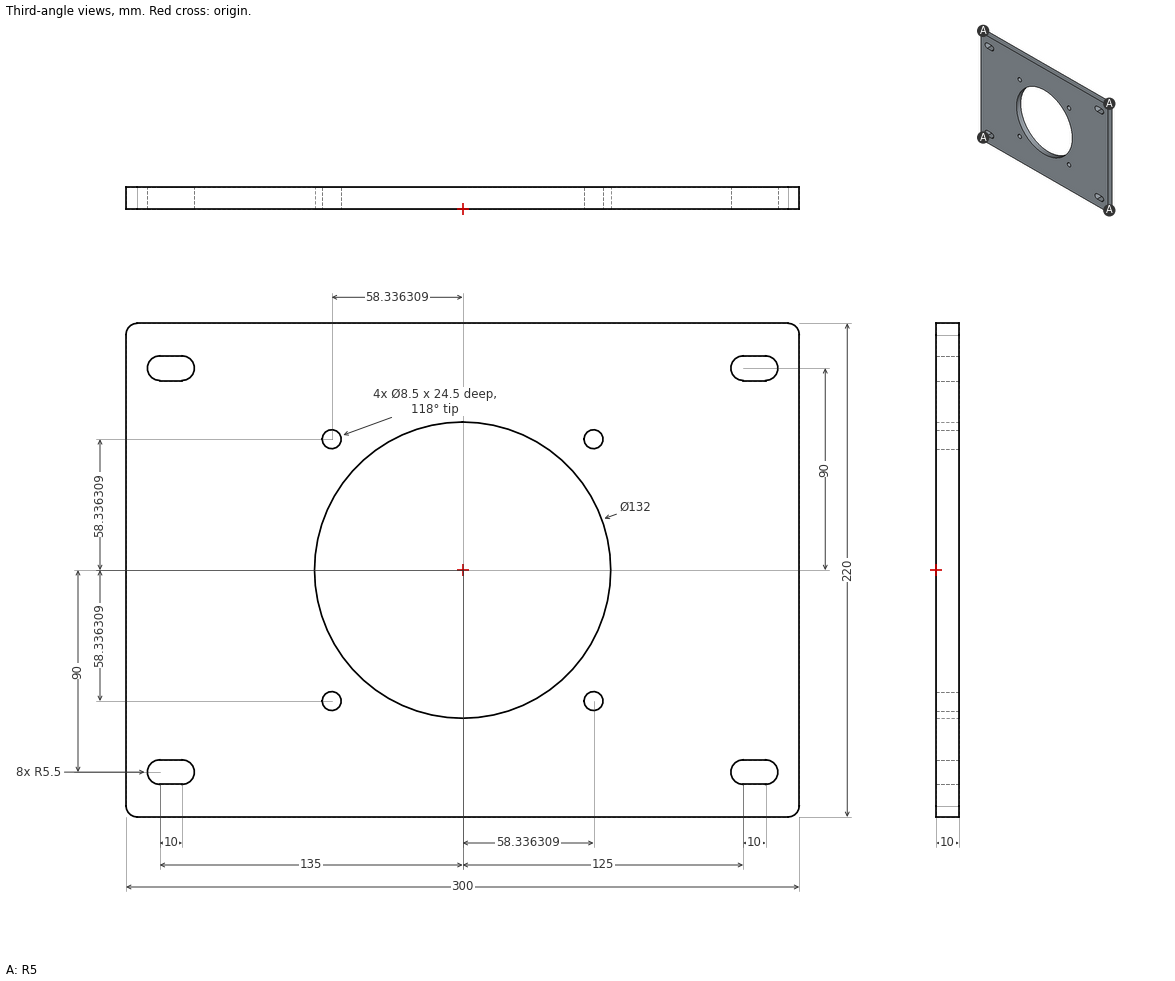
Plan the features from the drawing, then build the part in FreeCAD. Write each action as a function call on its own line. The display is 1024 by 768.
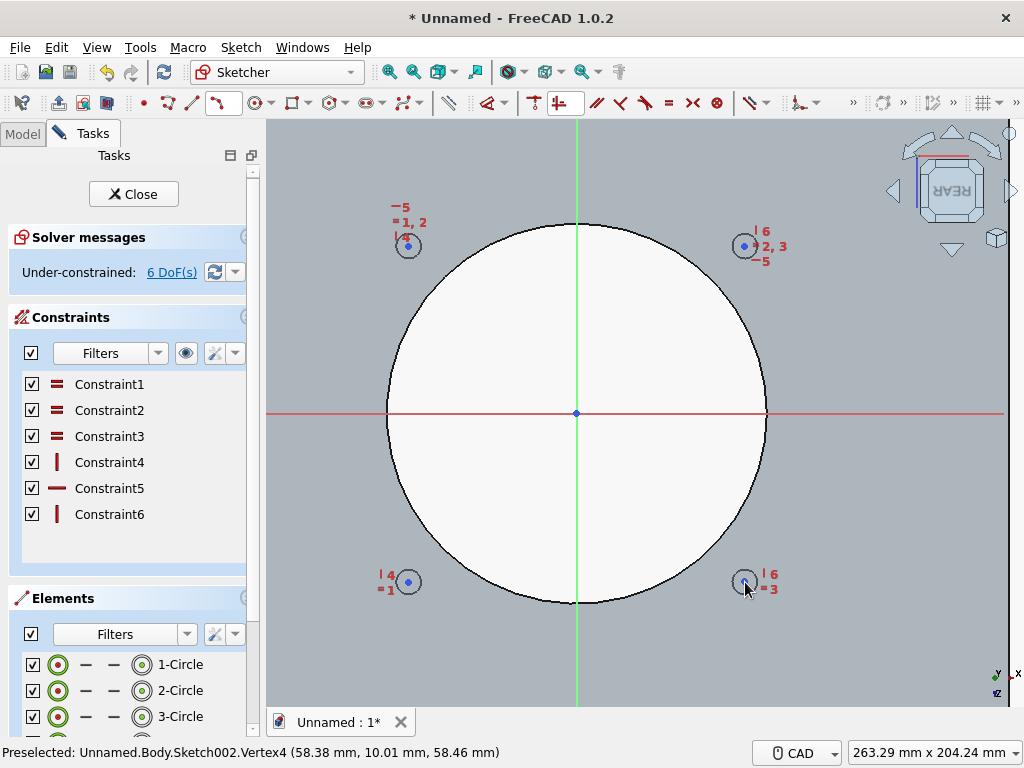
click(409, 582)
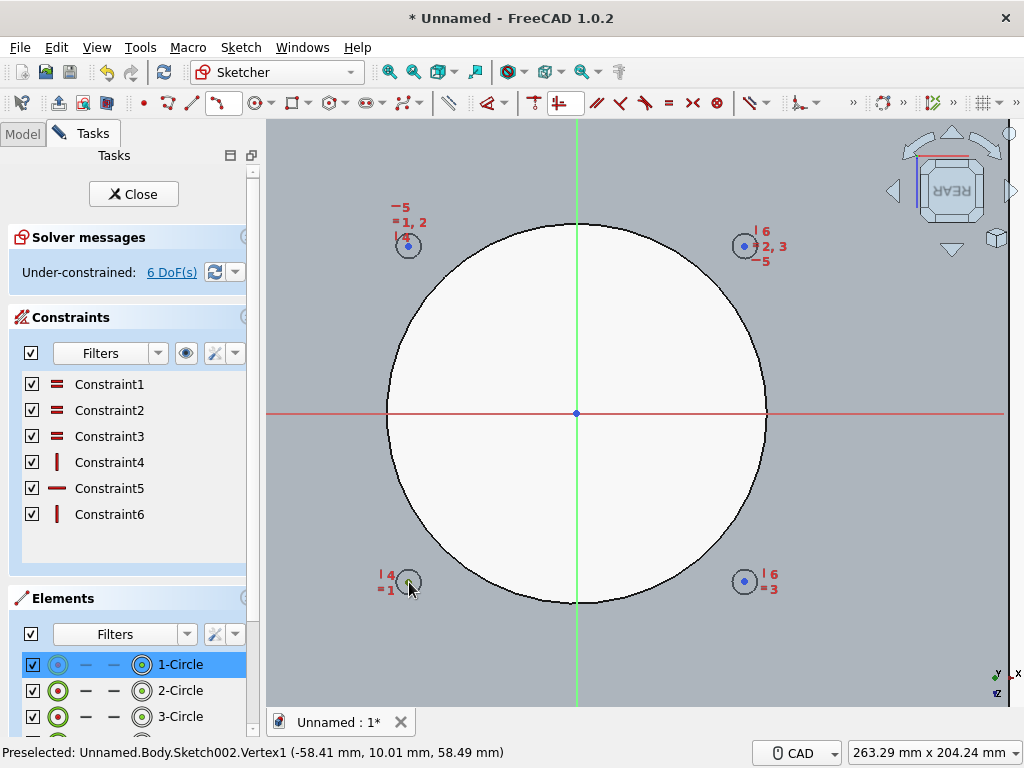
click(745, 582)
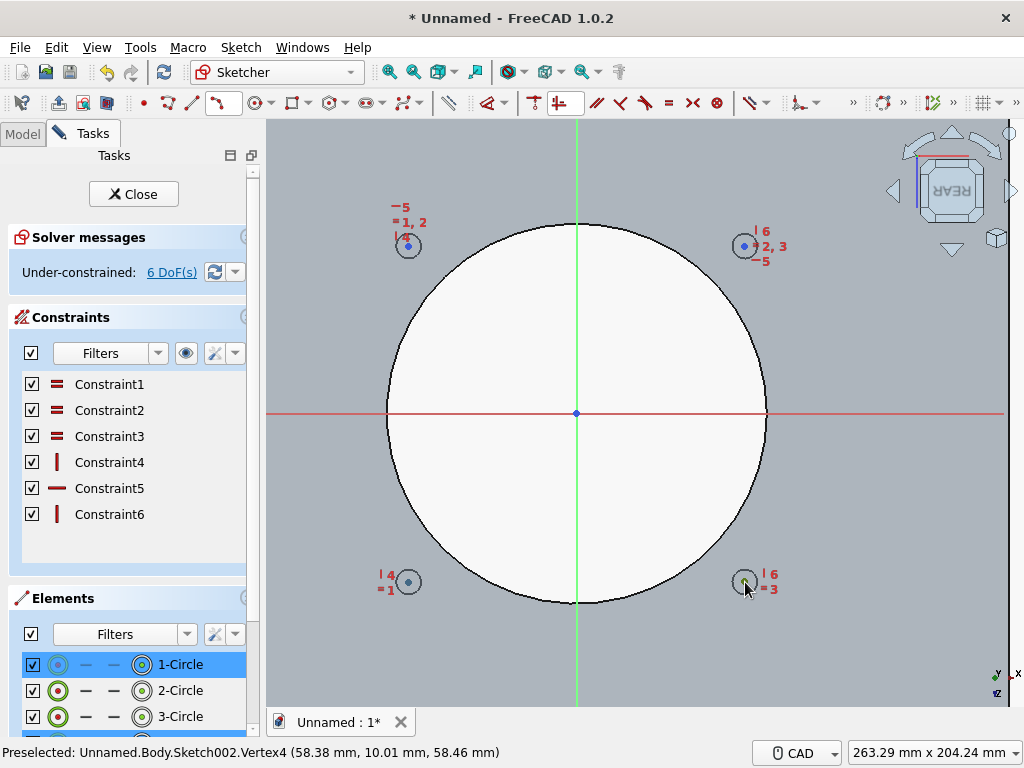
key(h)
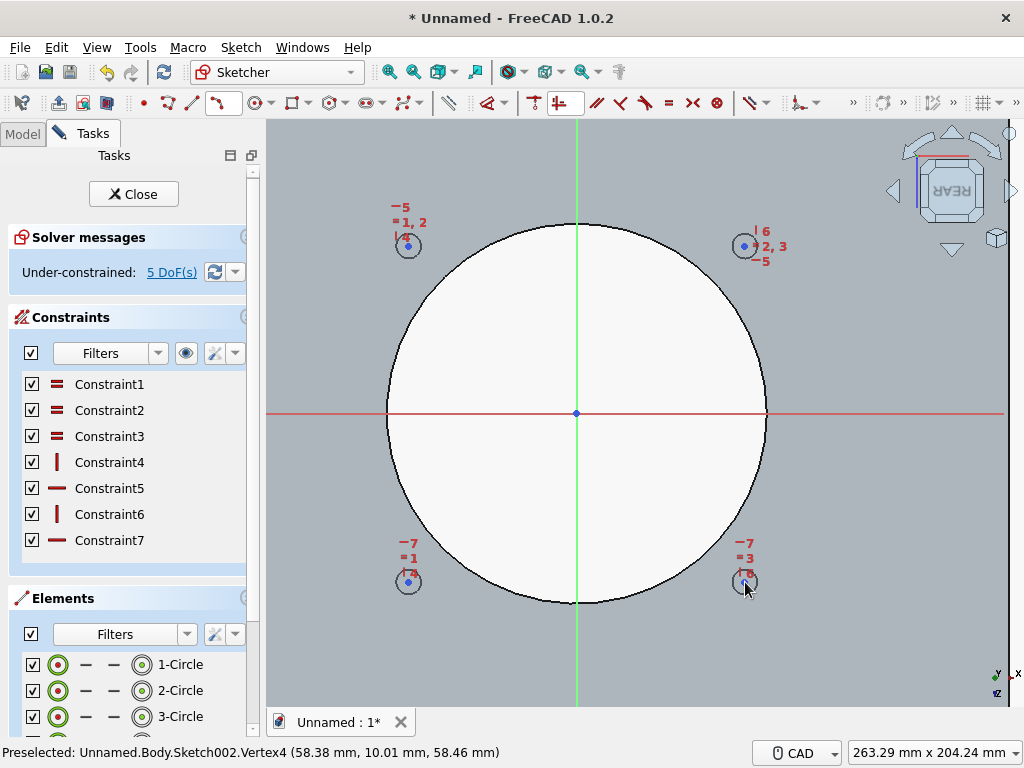
key(d)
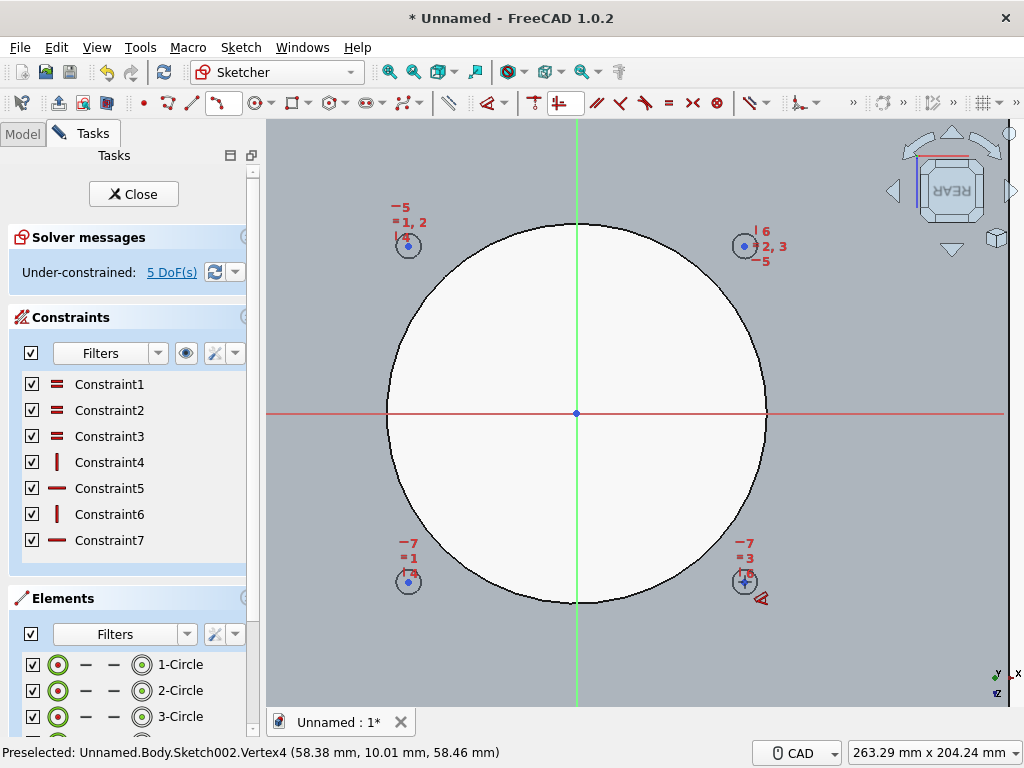
scroll(417, 573, up, 3)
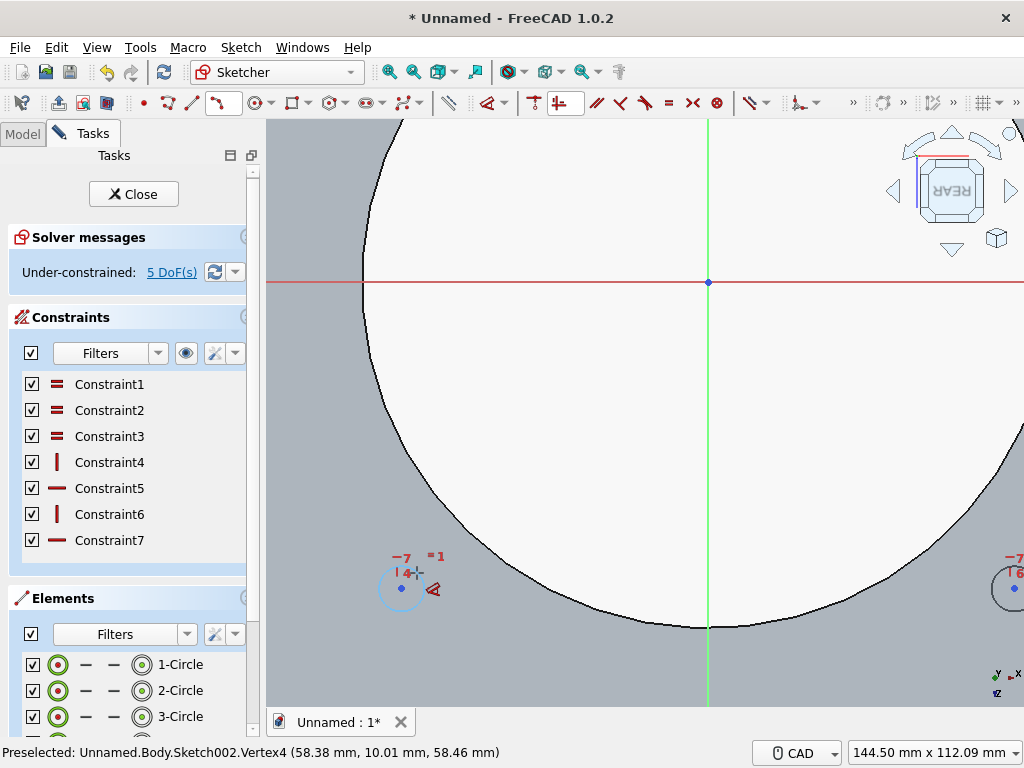
click(418, 573)
click(441, 551)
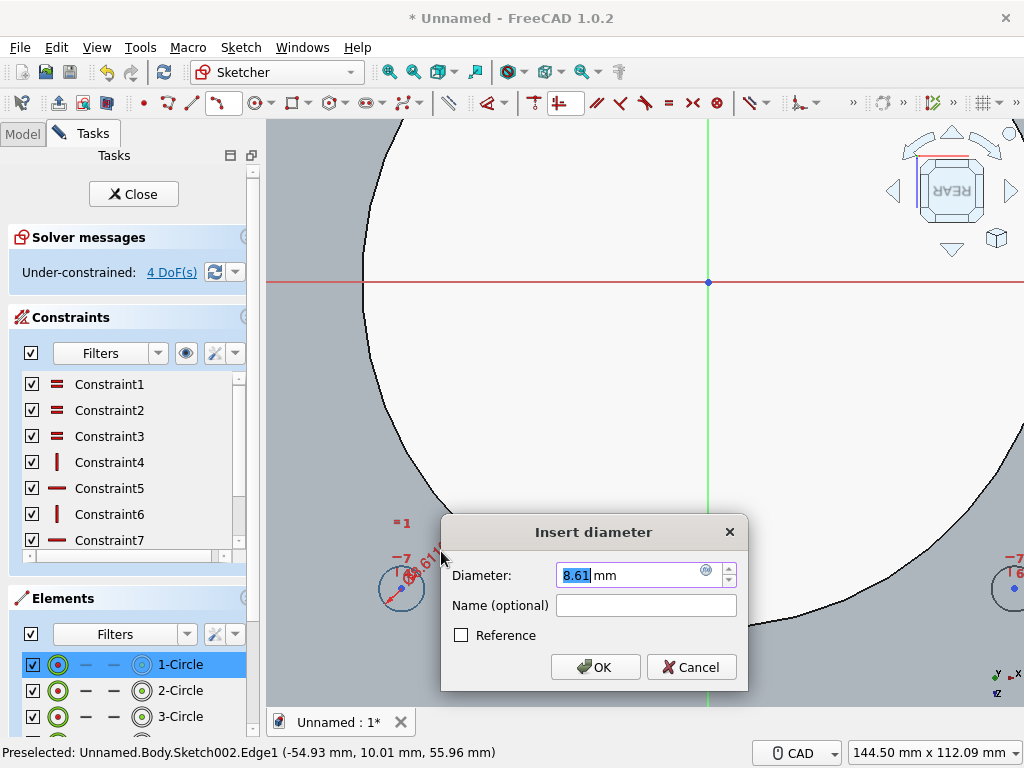
text(8.5)
key(Return)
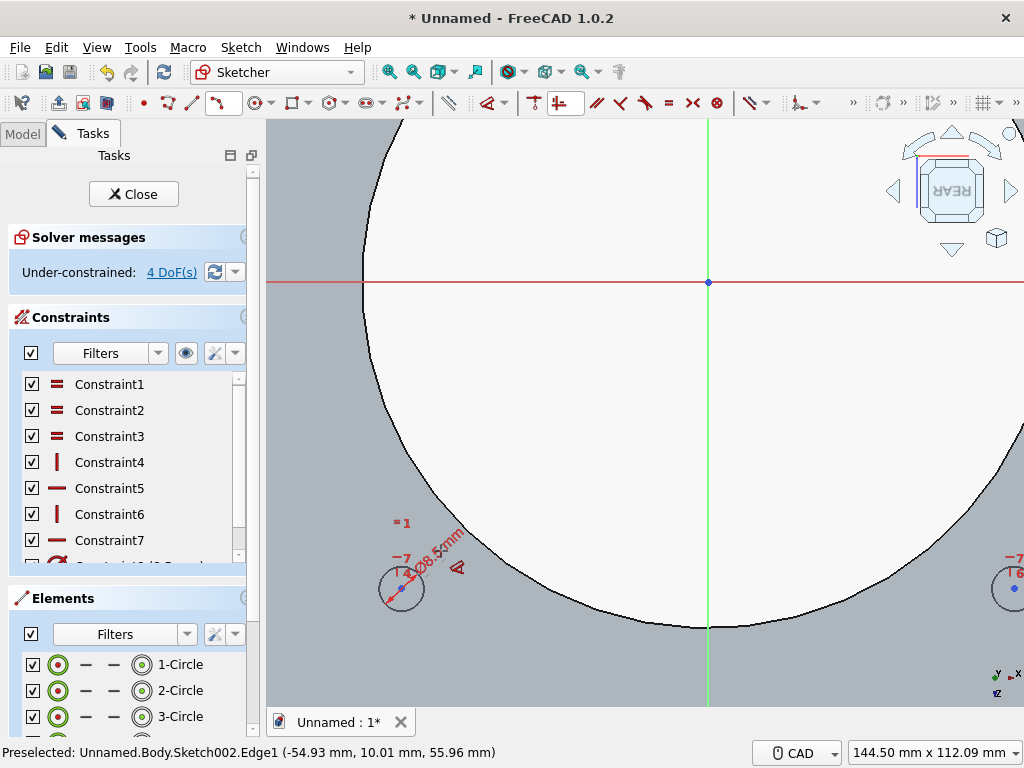
click(402, 589)
click(555, 623)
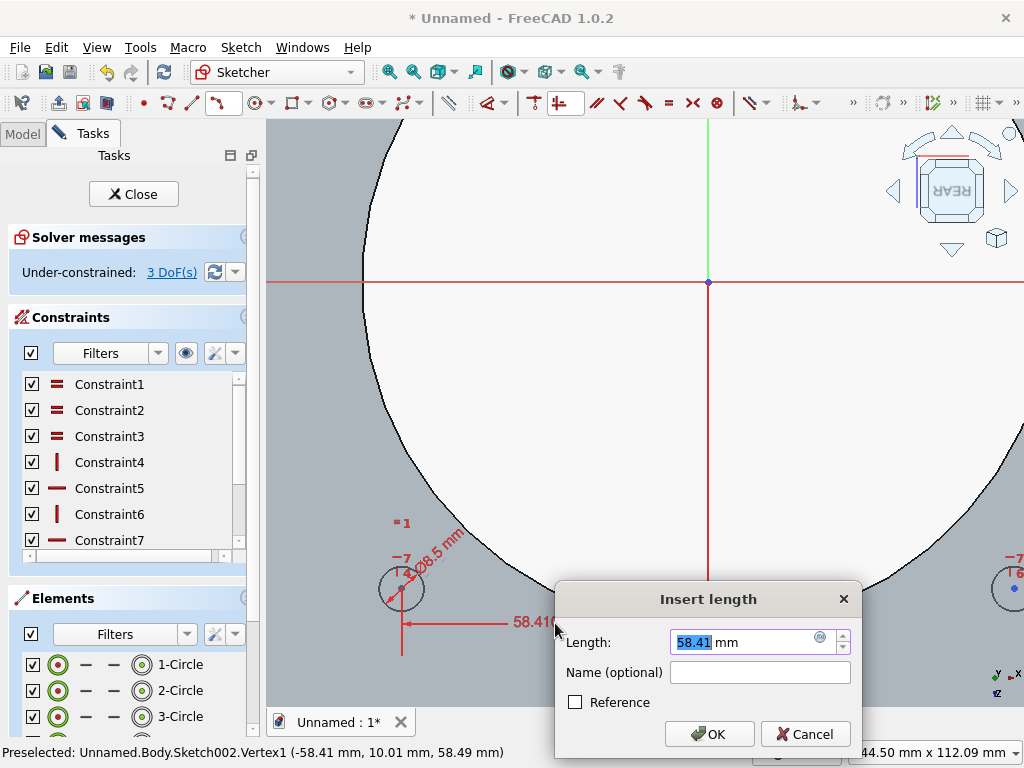
text(58.336309)
key(Return)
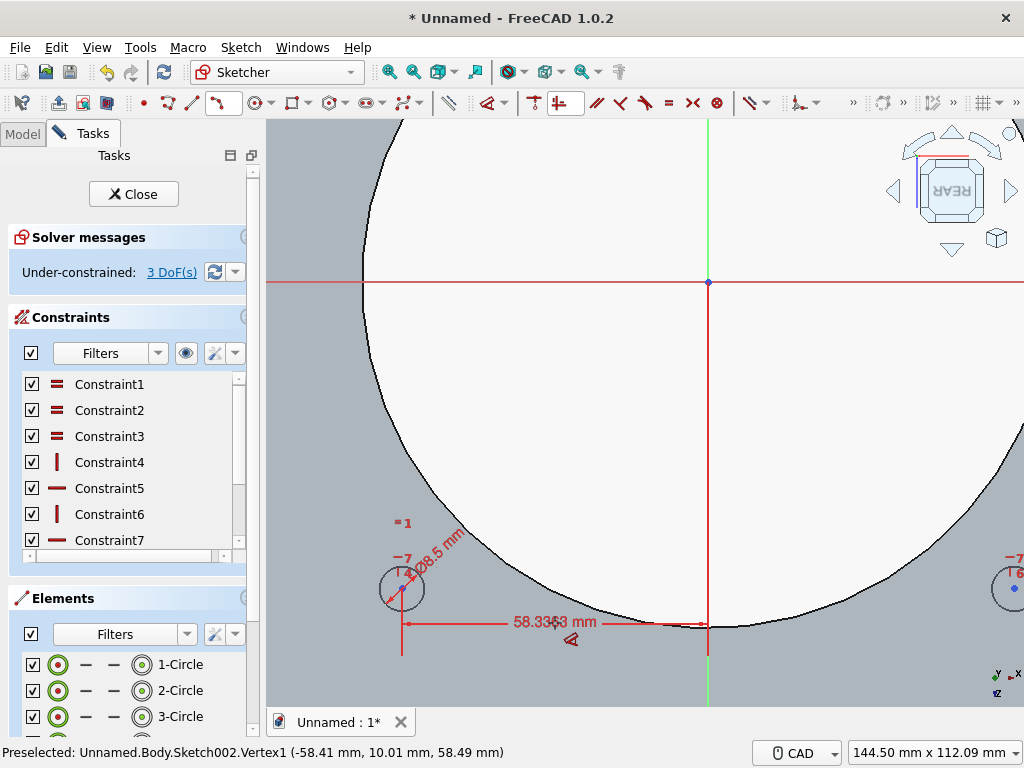
click(402, 589)
click(368, 436)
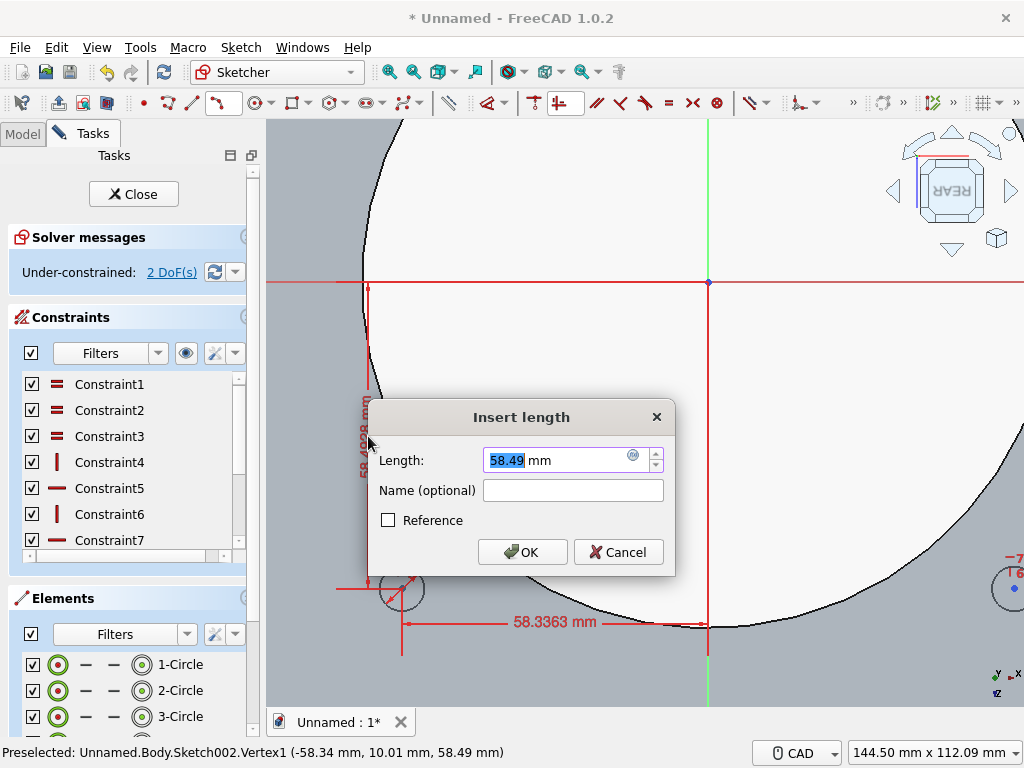
text(58.336309)
key(Return)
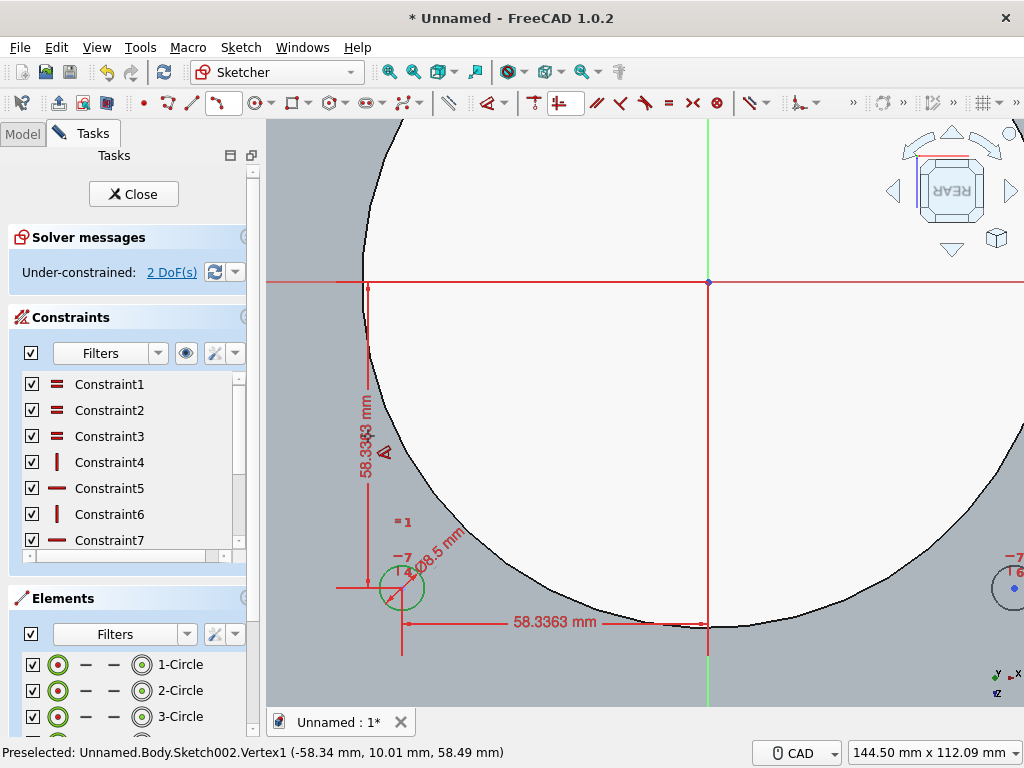
scroll(417, 572, down, 3)